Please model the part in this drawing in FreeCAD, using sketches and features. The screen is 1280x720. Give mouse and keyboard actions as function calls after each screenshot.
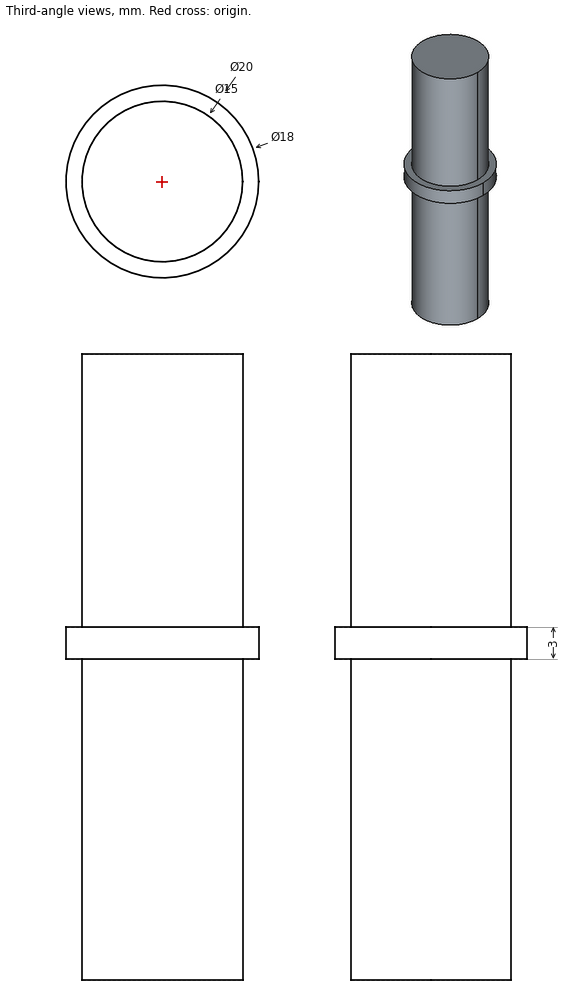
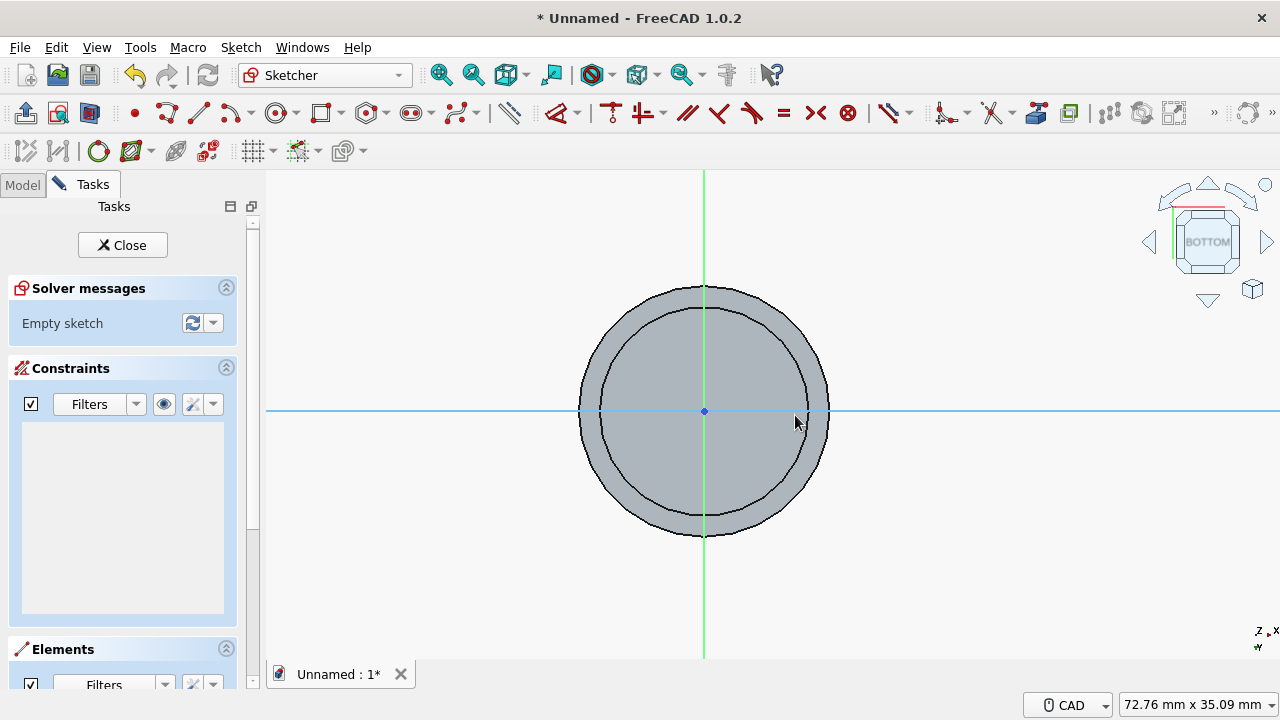
key(g)
key(c)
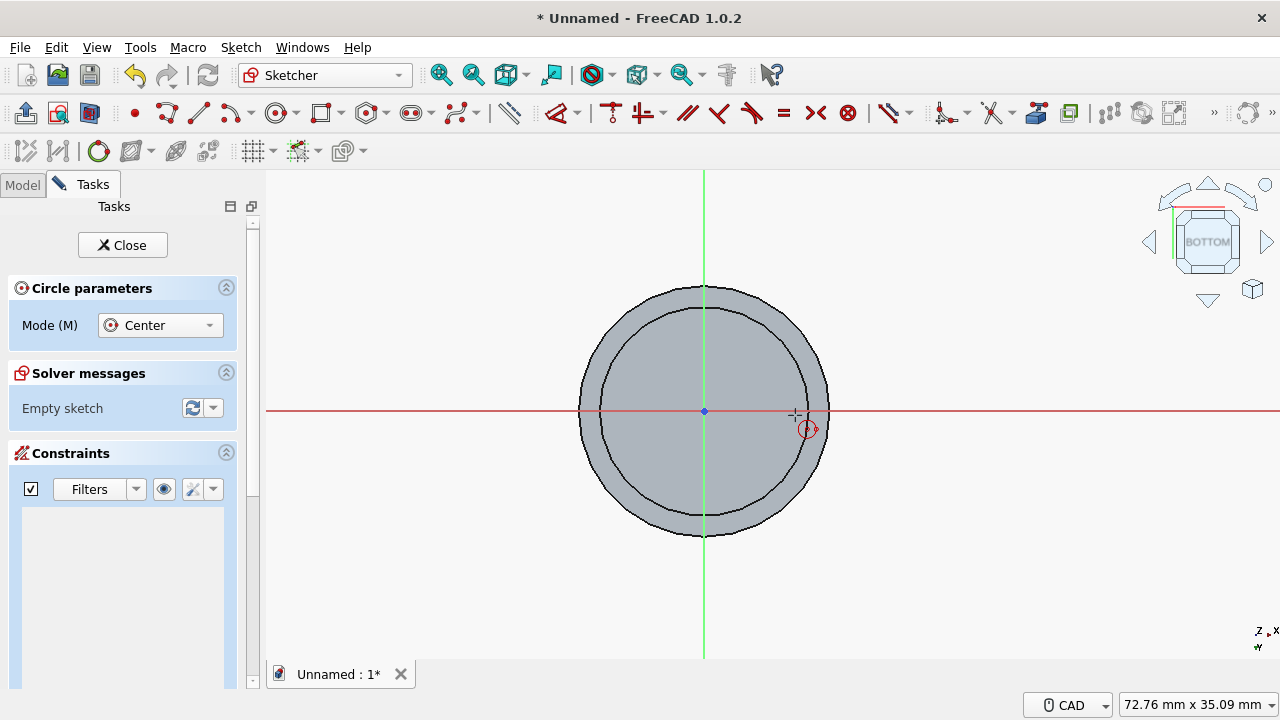
click(704, 411)
click(803, 313)
key(Escape)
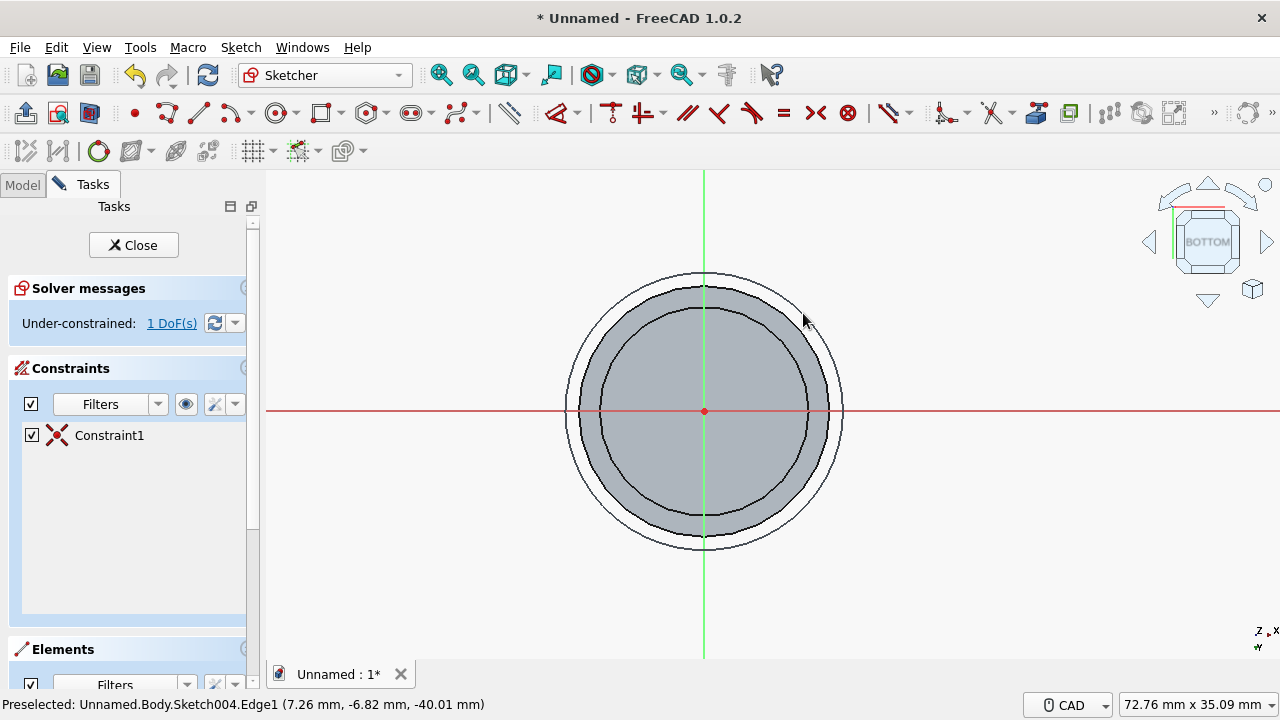
key(d)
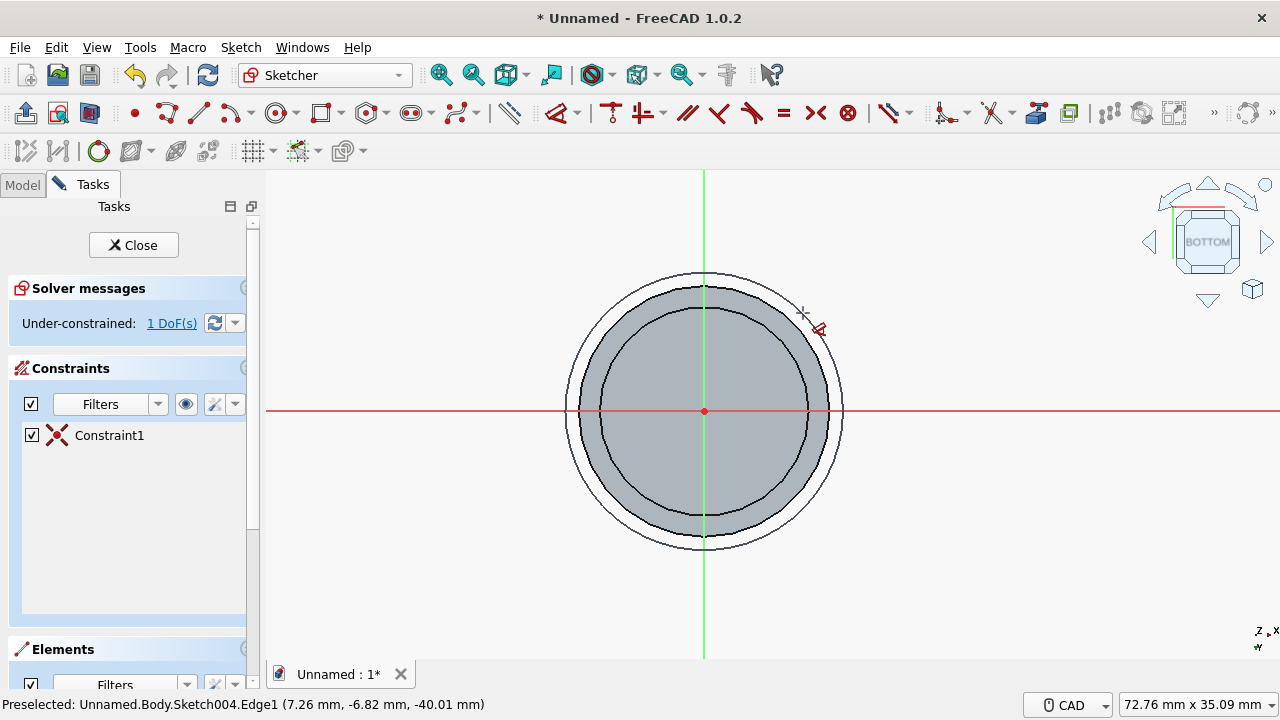
click(802, 313)
click(825, 290)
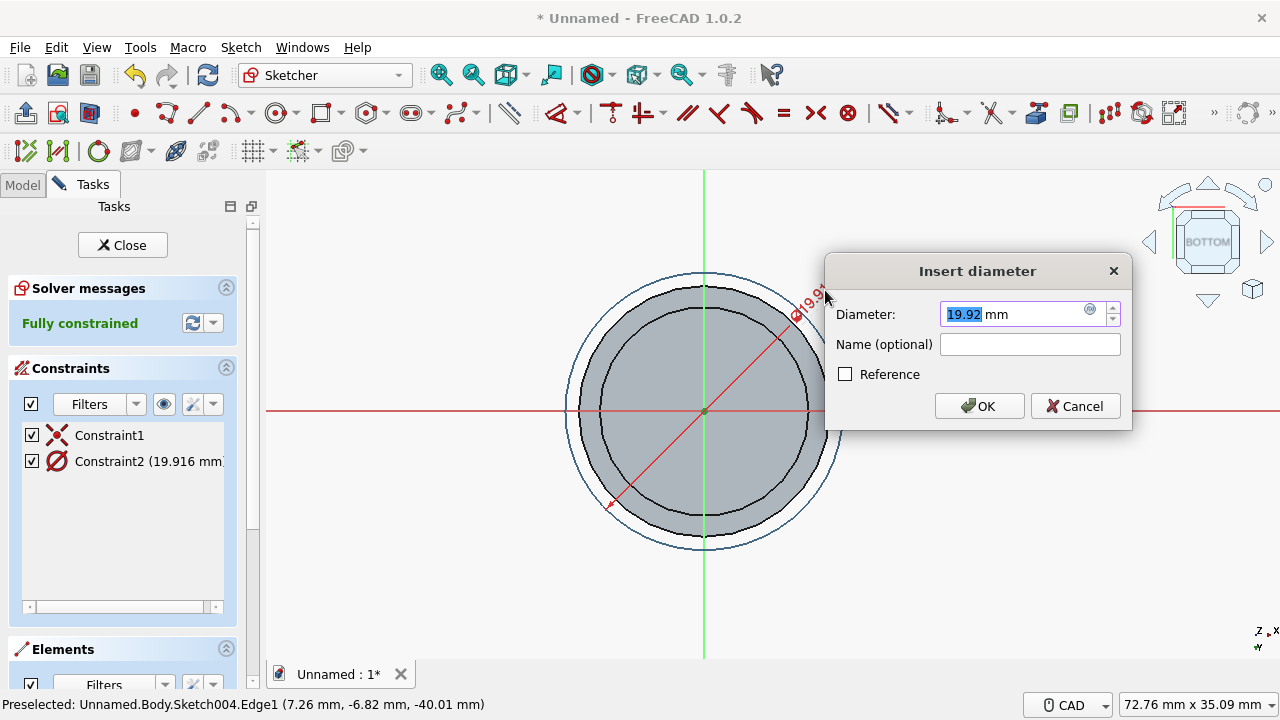
text(20)
key(Return)
key(Escape)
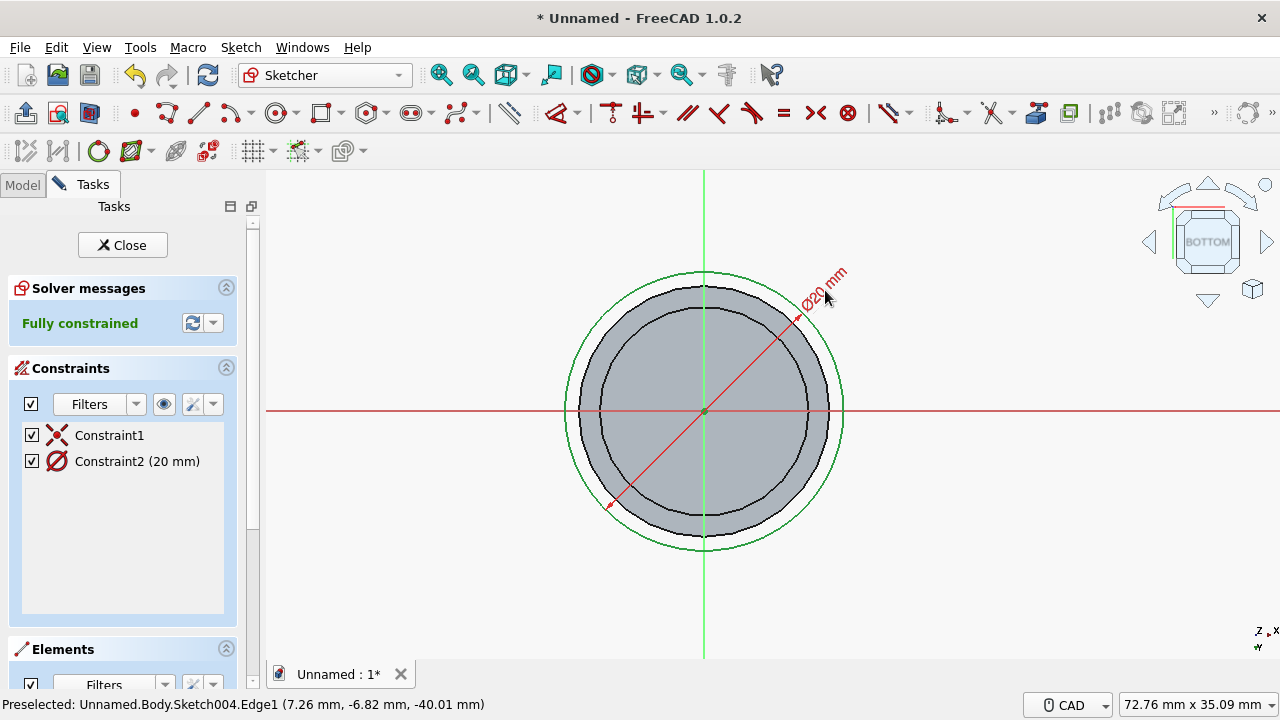
click(123, 245)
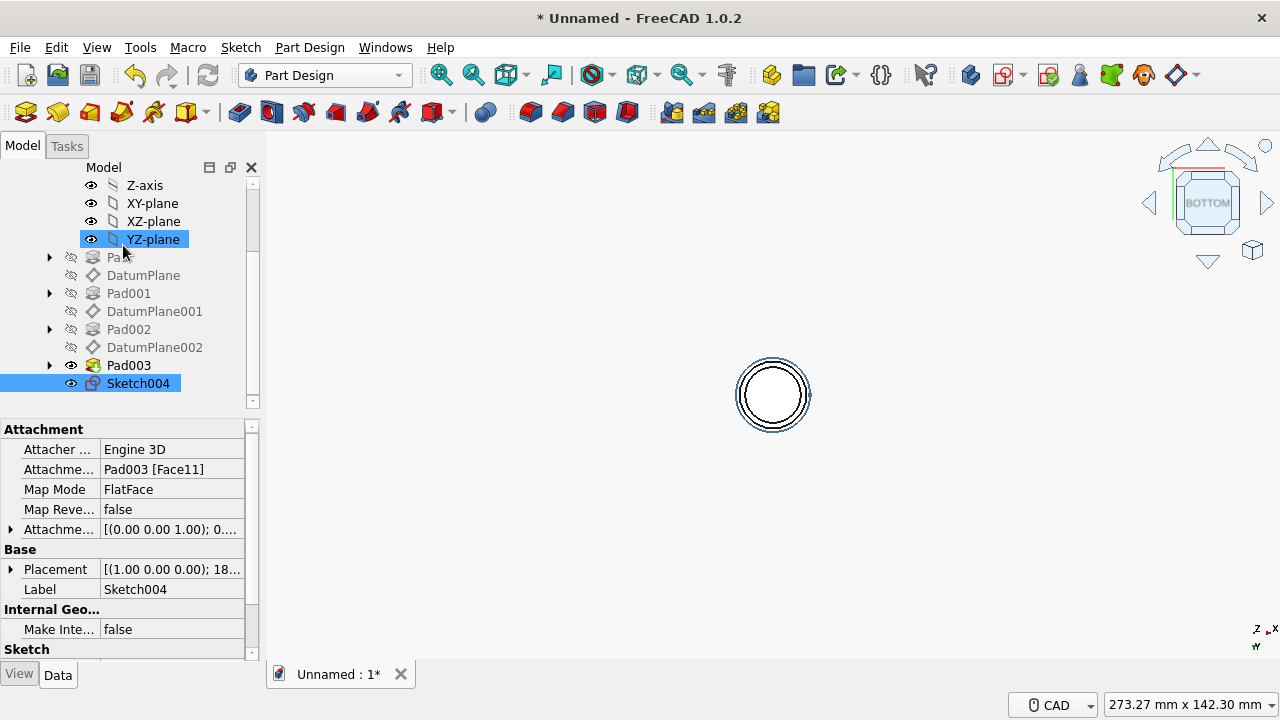
click(240, 112)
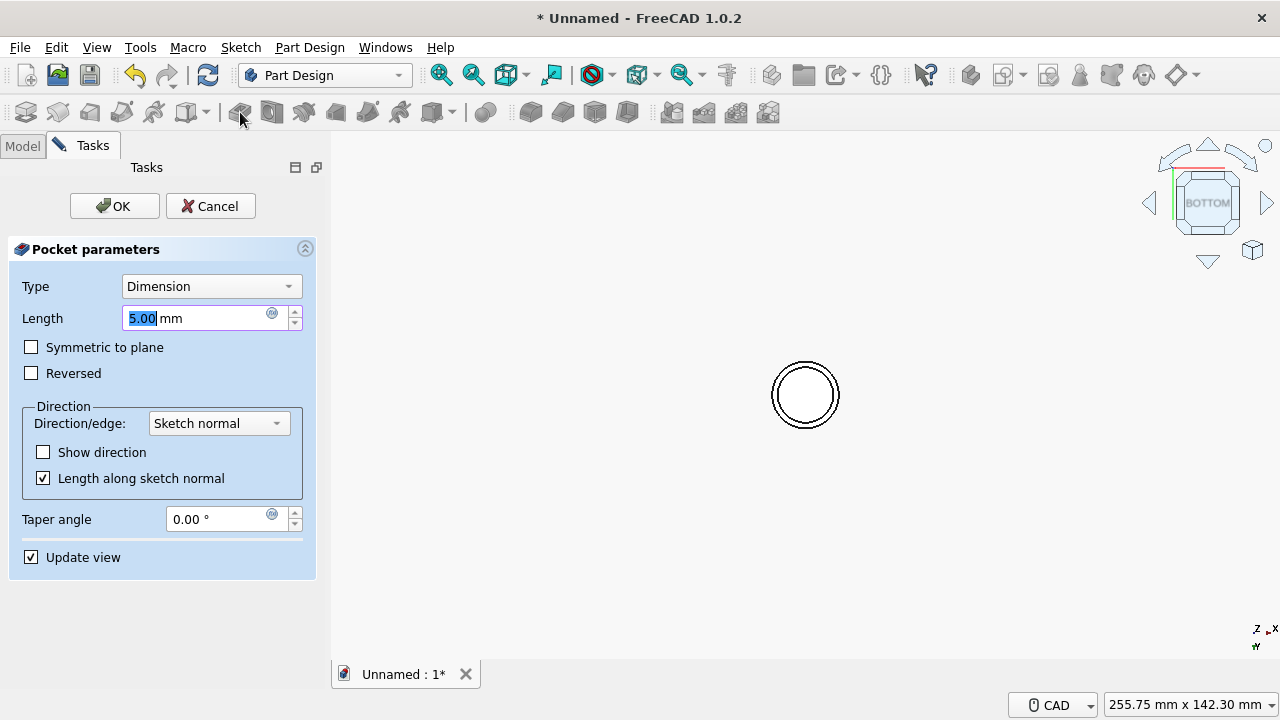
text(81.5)
key(Tab)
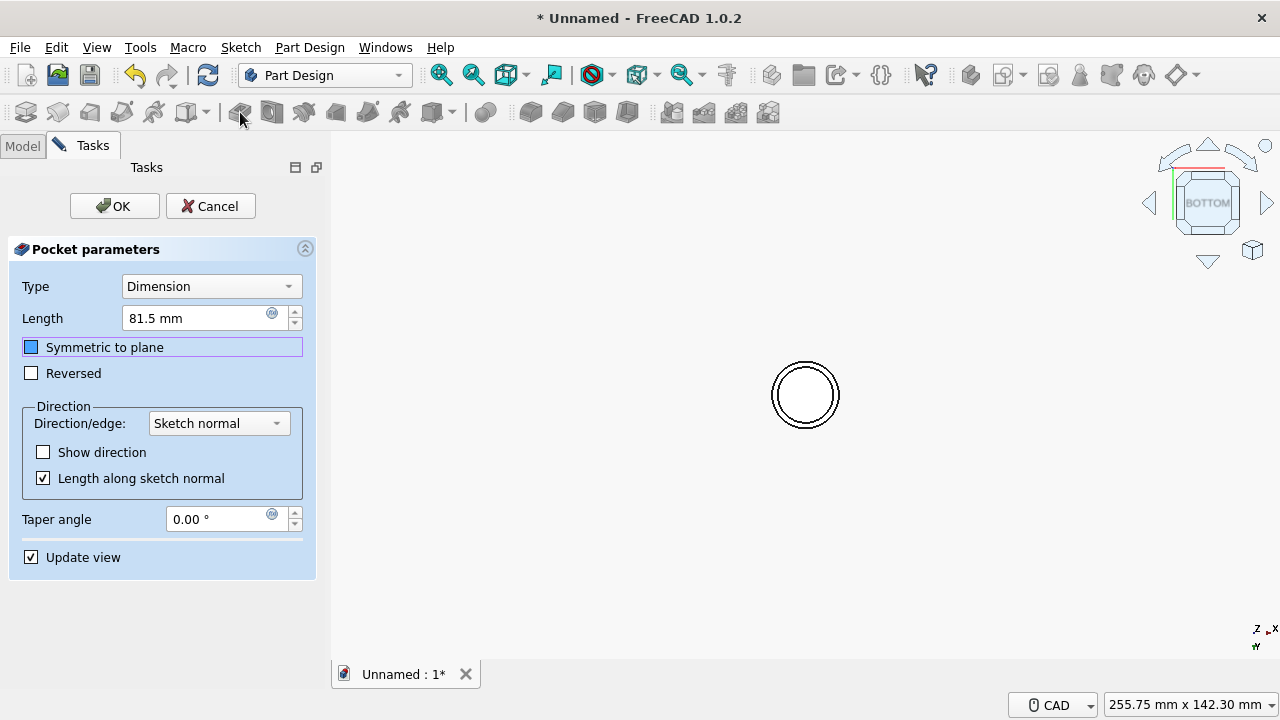
click(115, 206)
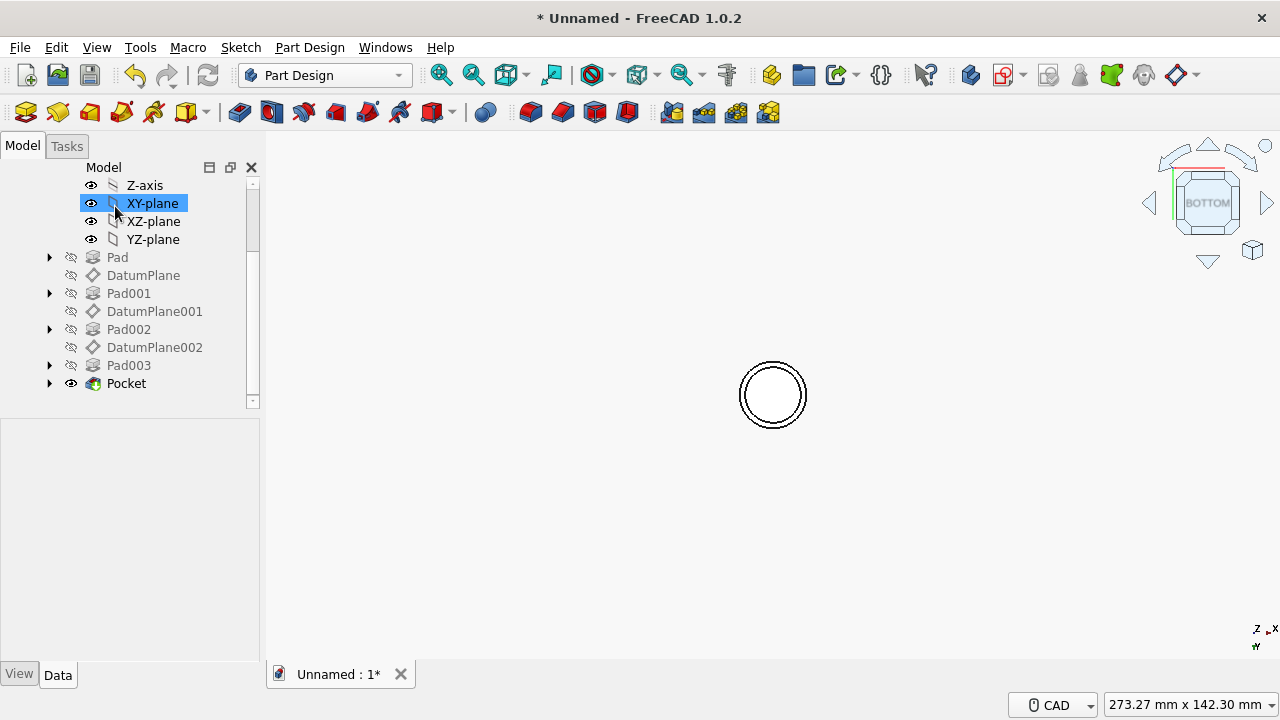
key(0)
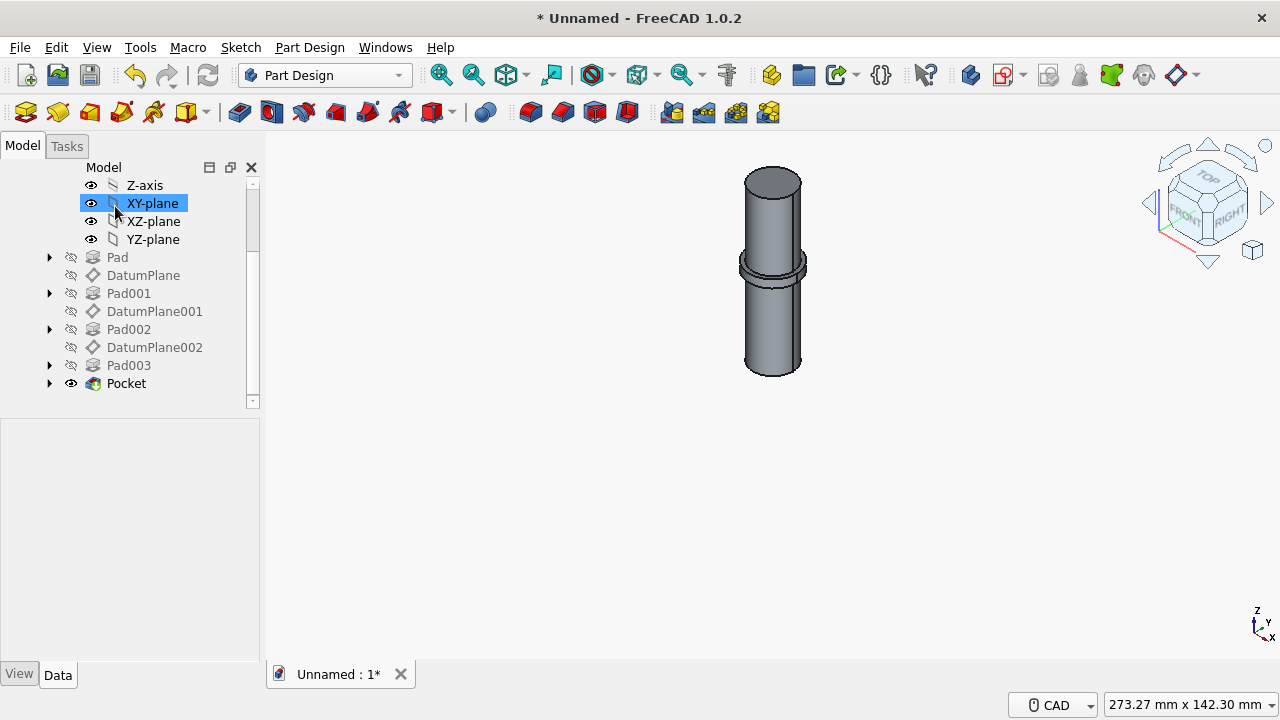
click(442, 76)